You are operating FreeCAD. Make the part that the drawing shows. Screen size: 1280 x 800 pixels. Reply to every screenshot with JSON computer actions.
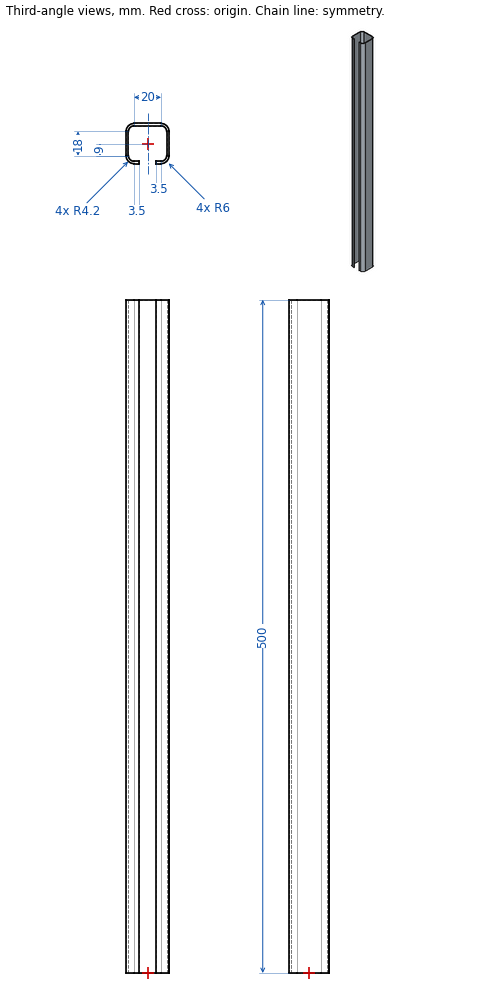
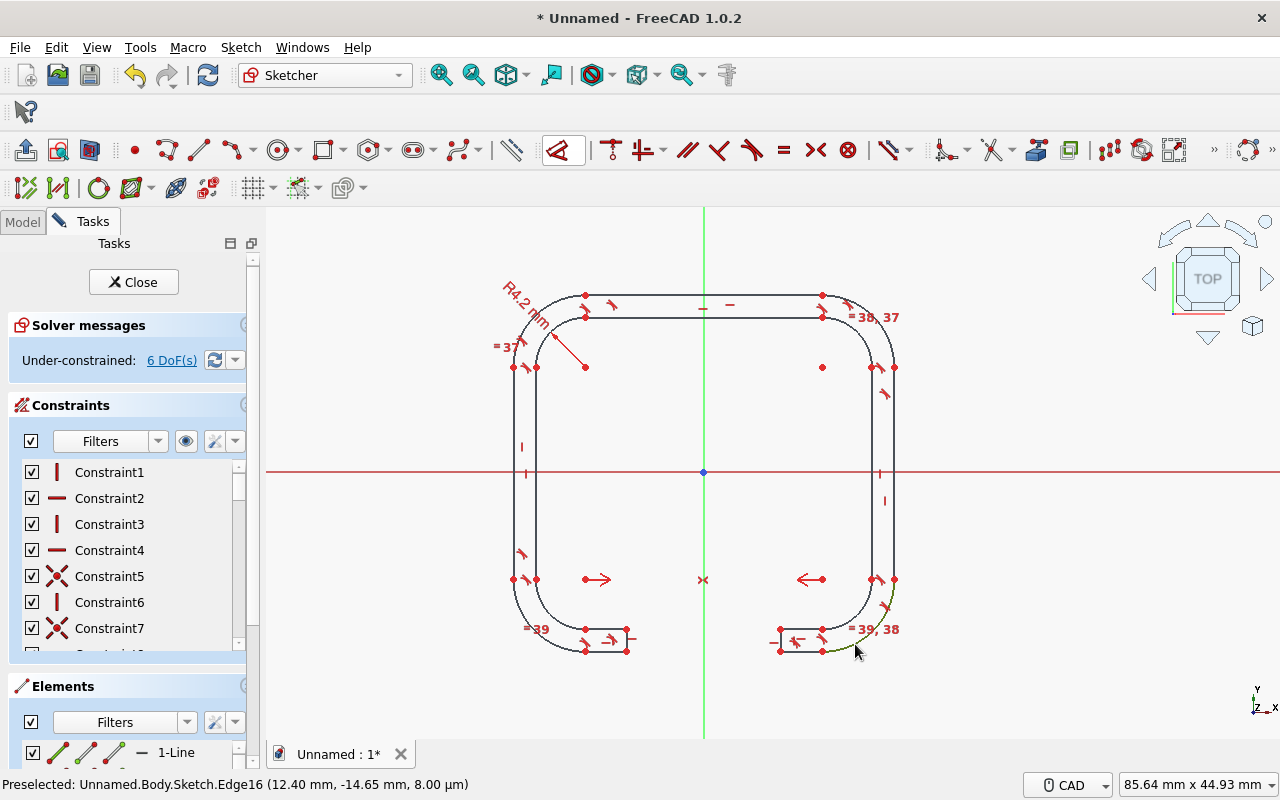
{"action": "left_click", "coordinate": [580, 150]}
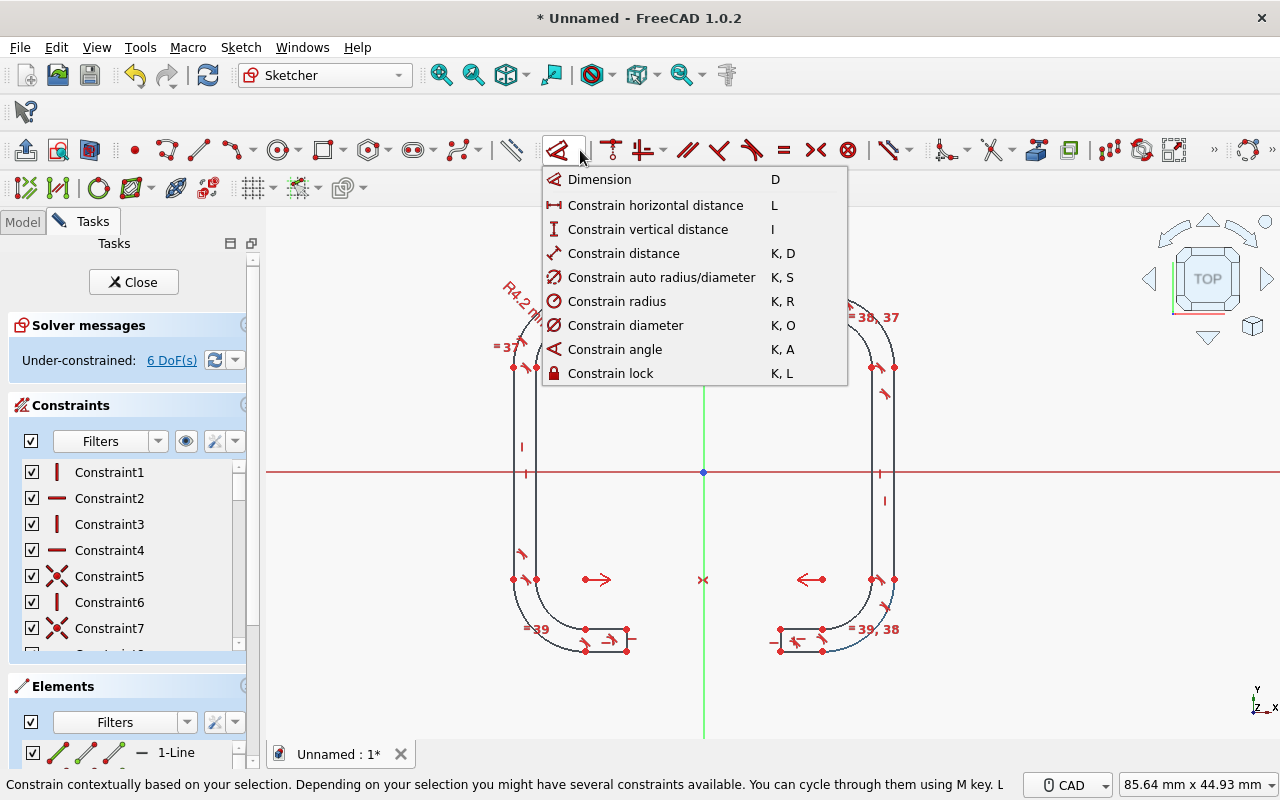
{"action": "left_click", "coordinate": [695, 301]}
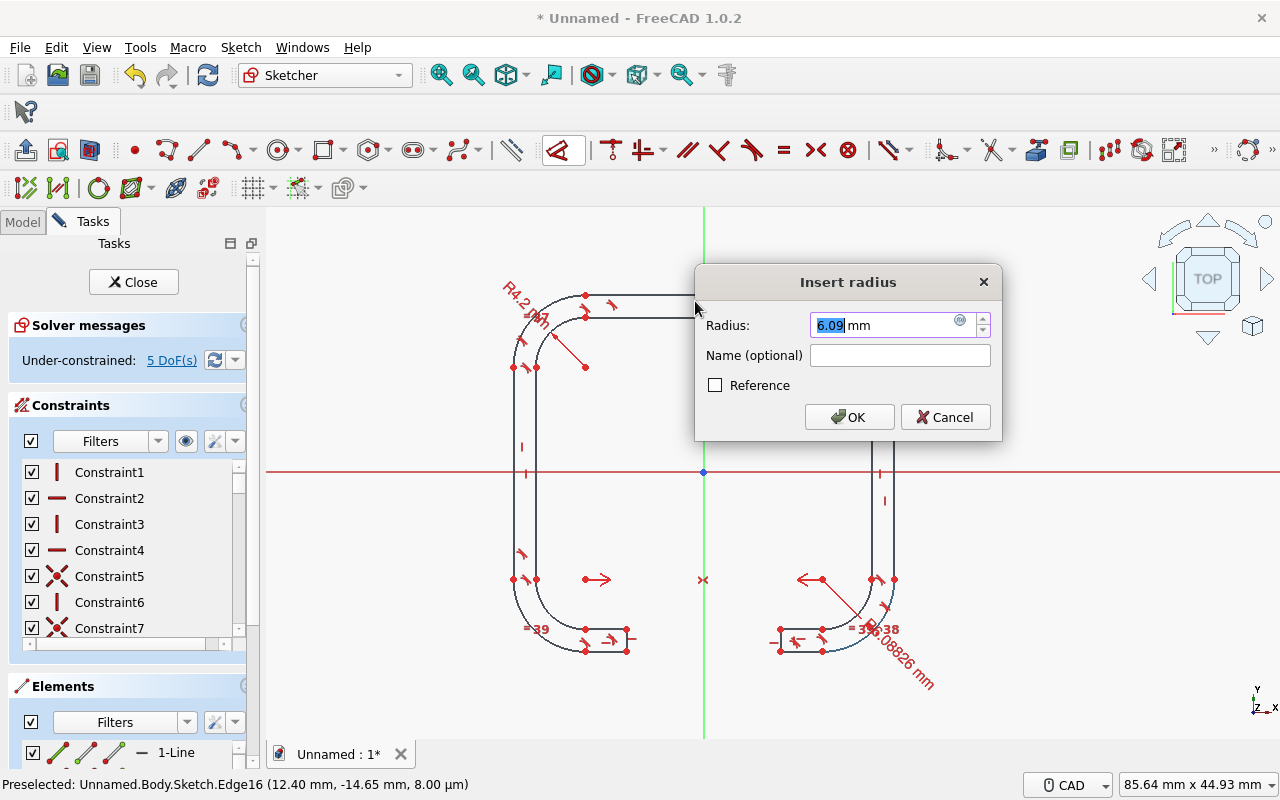
{"action": "type", "text": "6"}
{"action": "key", "text": "Return"}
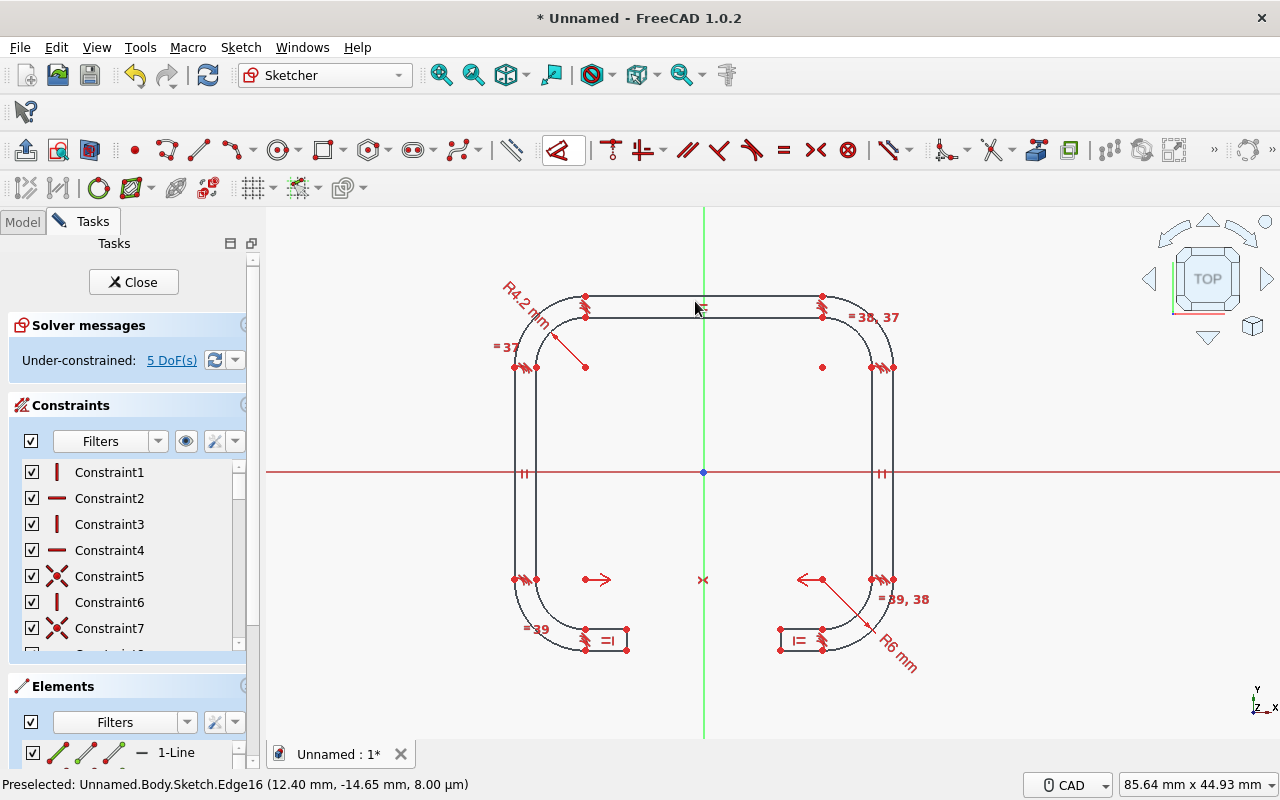
{"action": "left_click", "coordinate": [536, 516]}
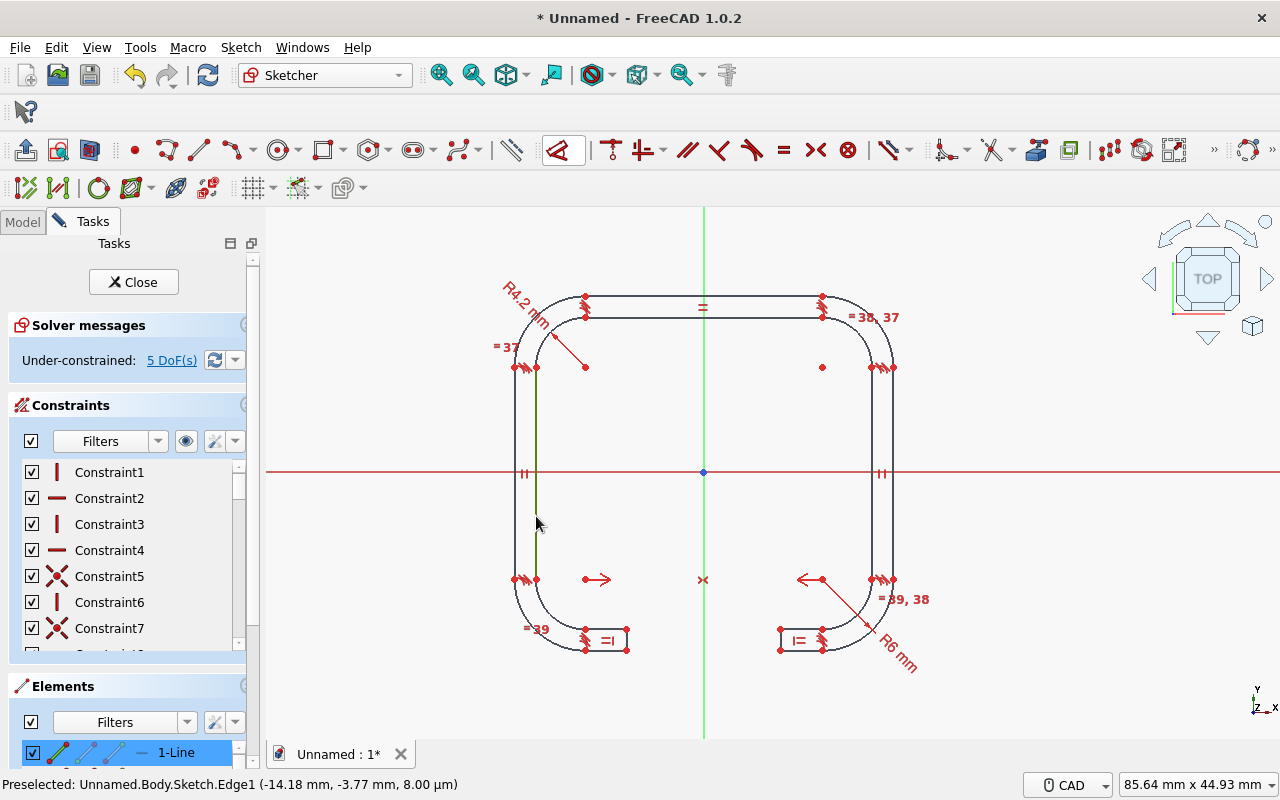
{"action": "key", "text": "i"}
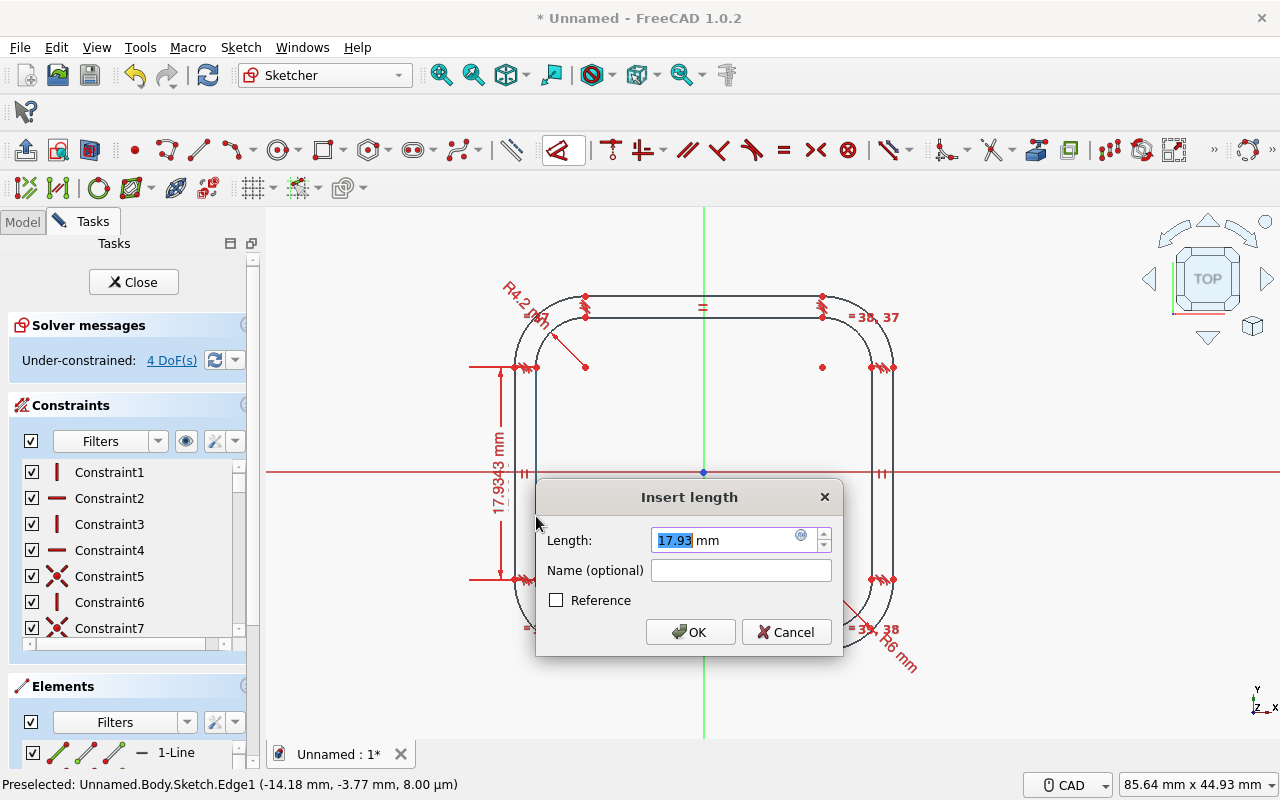
{"action": "type", "text": "18"}
{"action": "key", "text": "Return"}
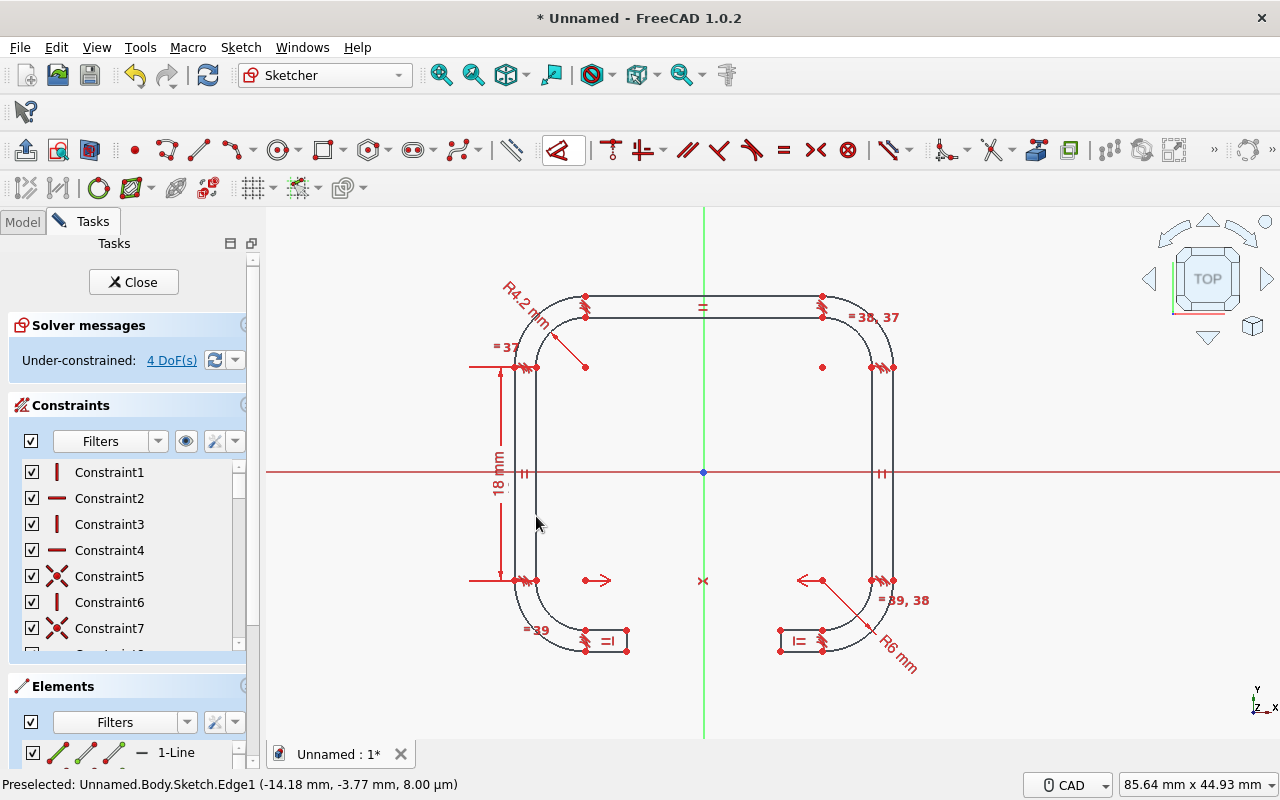
{"action": "left_click", "coordinate": [657, 318]}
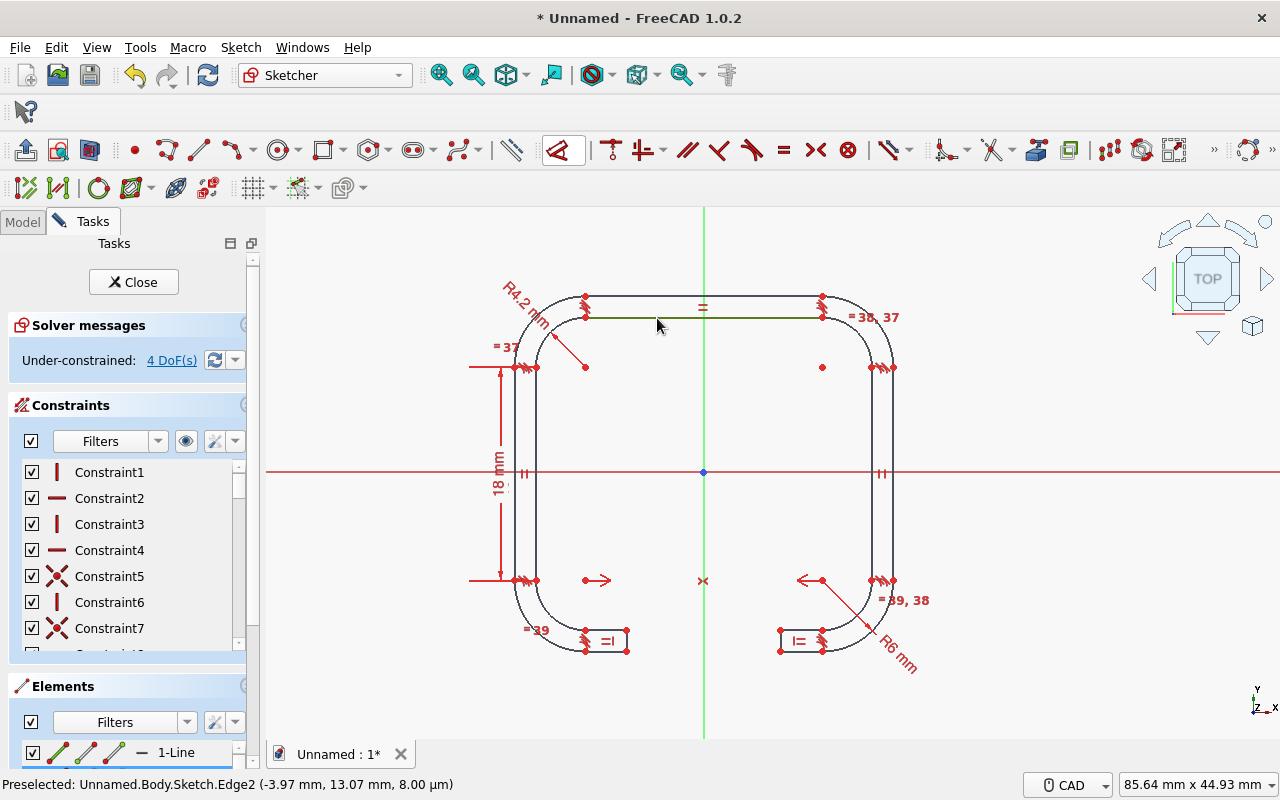
{"action": "left_click", "coordinate": [580, 150]}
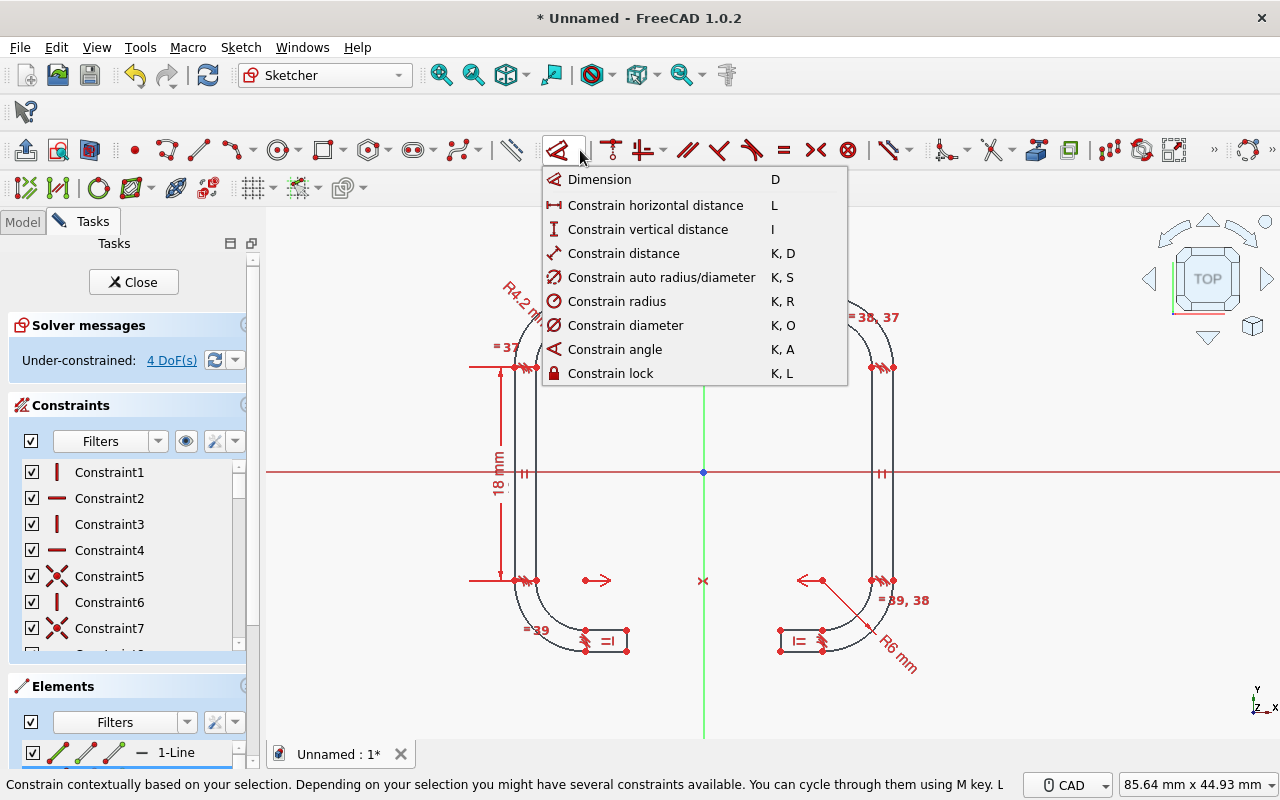
{"action": "left_click", "coordinate": [695, 205]}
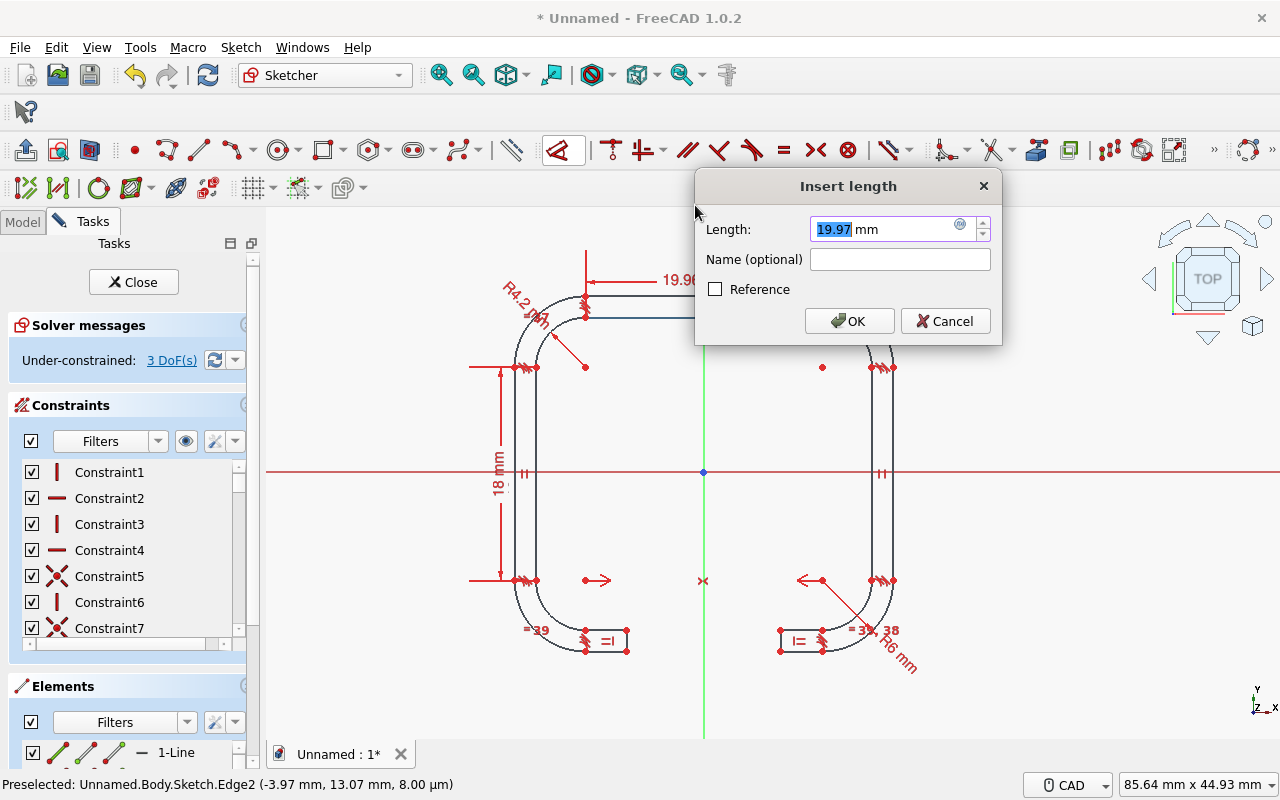
{"action": "type", "text": "20"}
{"action": "key", "text": "Return"}